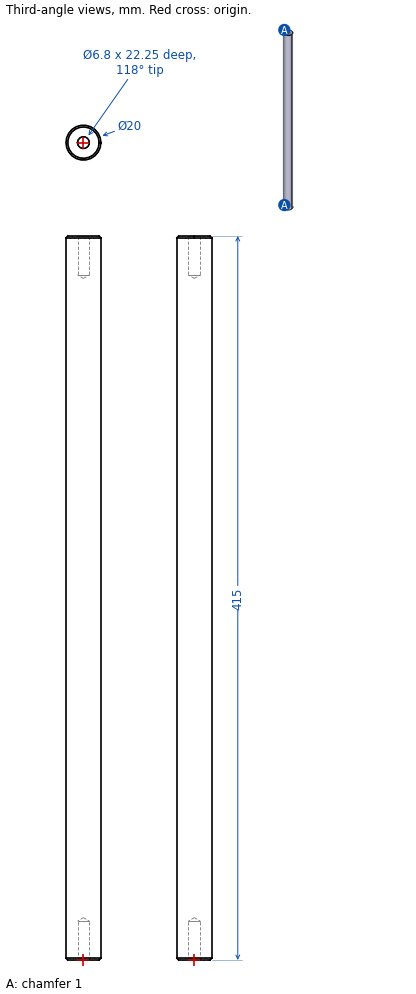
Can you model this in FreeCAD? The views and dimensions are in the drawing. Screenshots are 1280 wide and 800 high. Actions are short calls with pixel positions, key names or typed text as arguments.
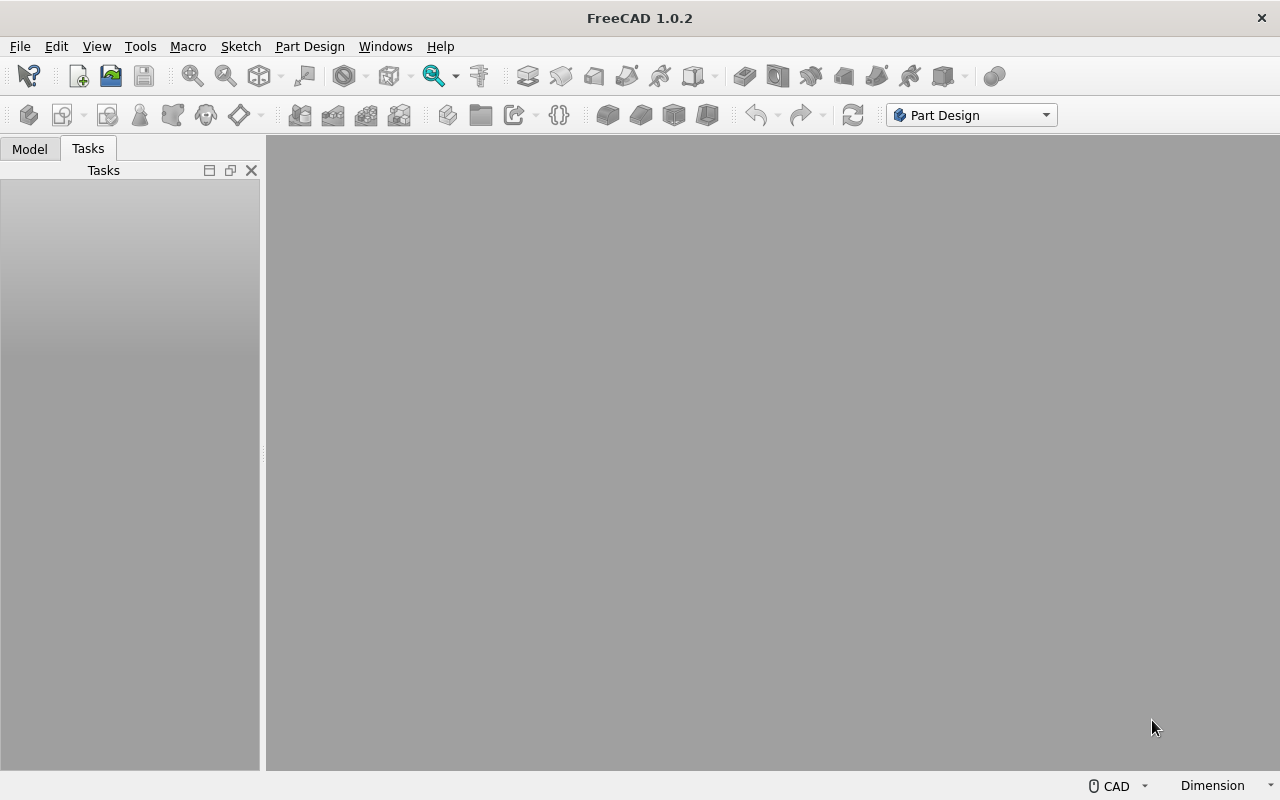
click(78, 76)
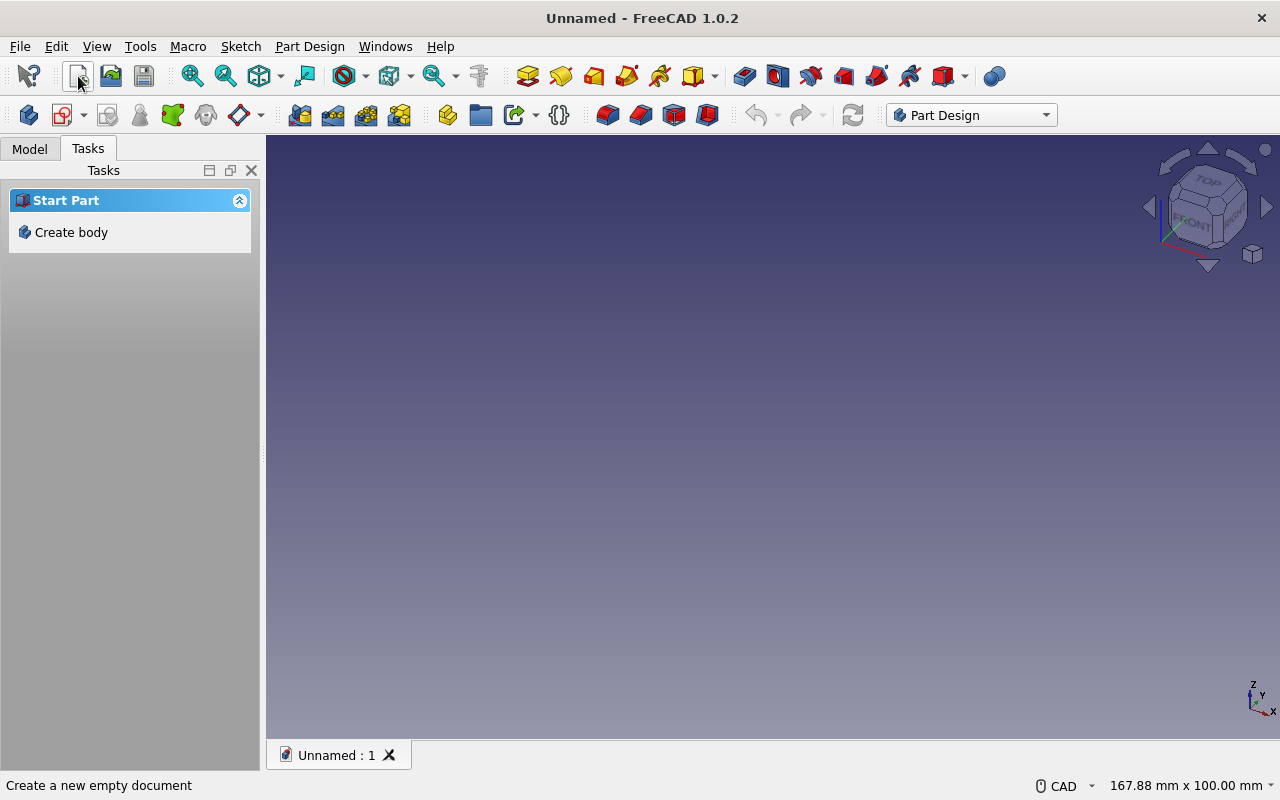
click(62, 116)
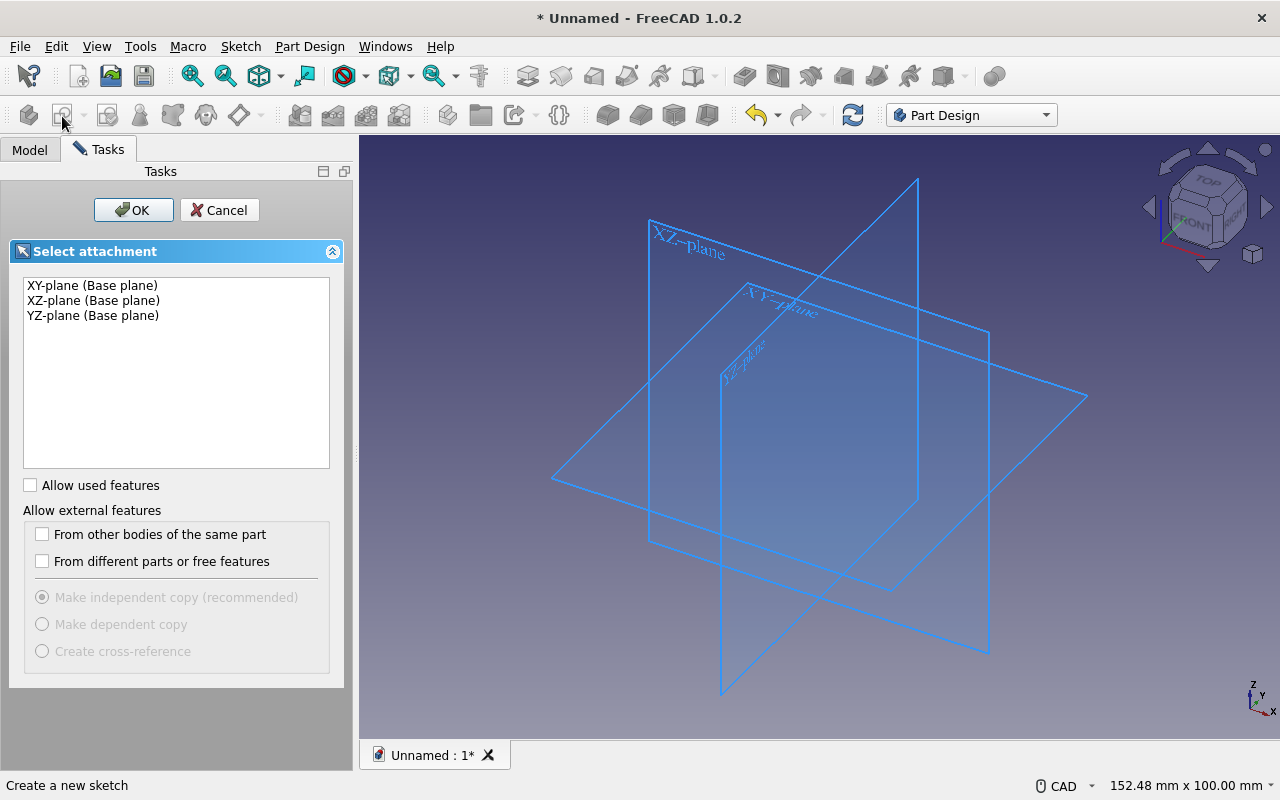
click(84, 286)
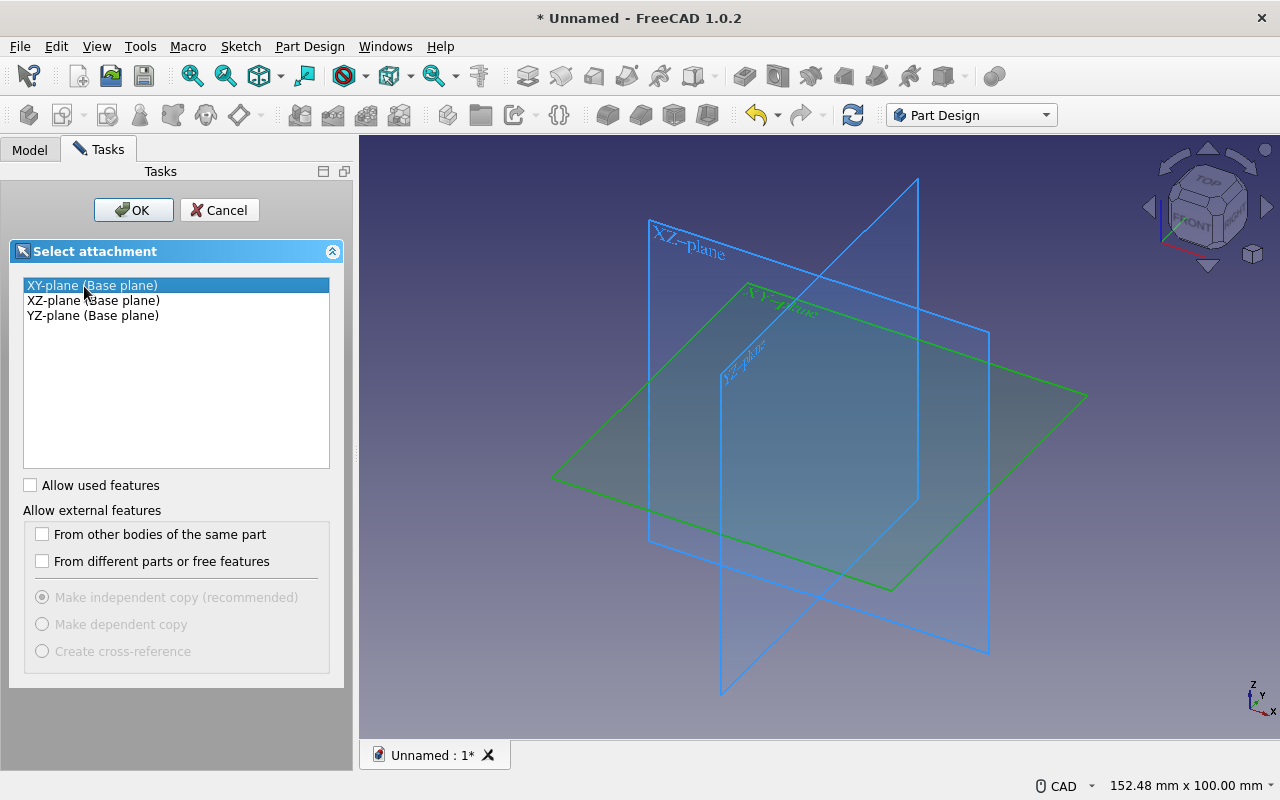
click(134, 210)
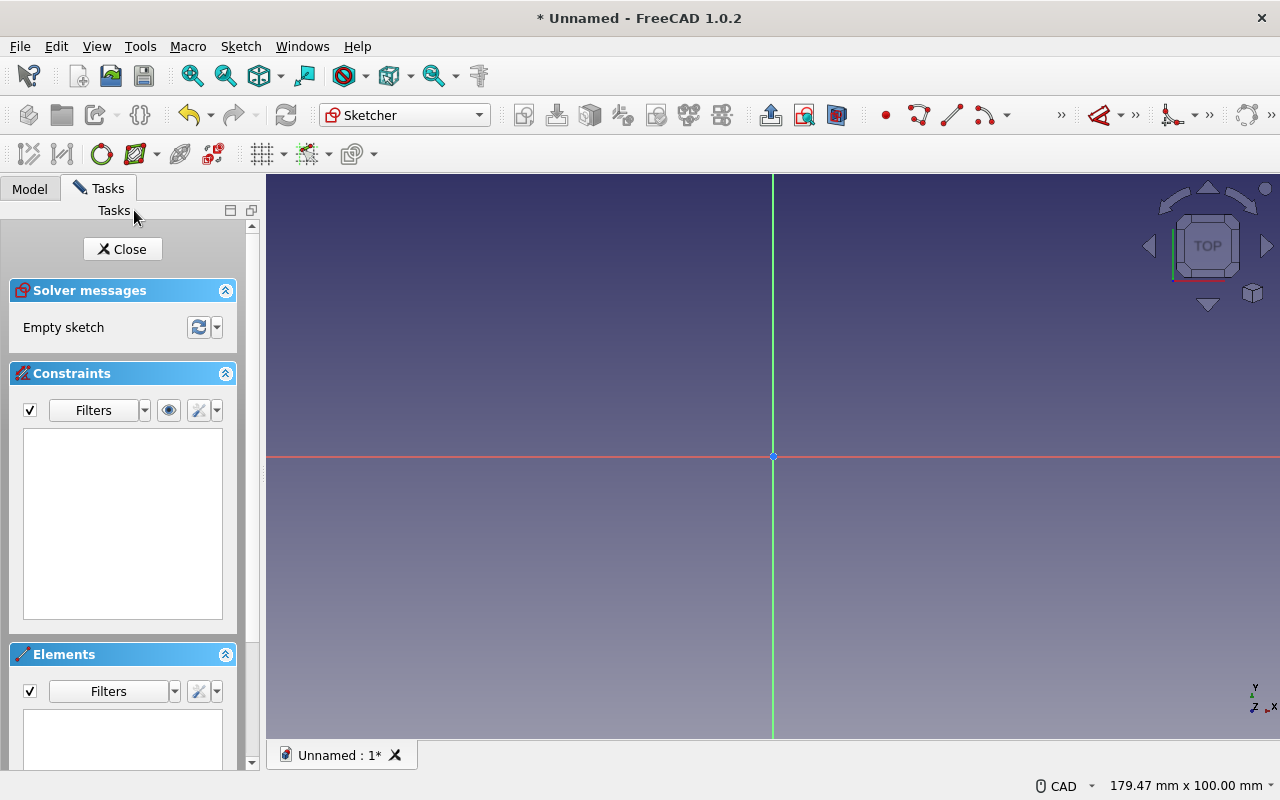
scroll(803, 456, up, 6)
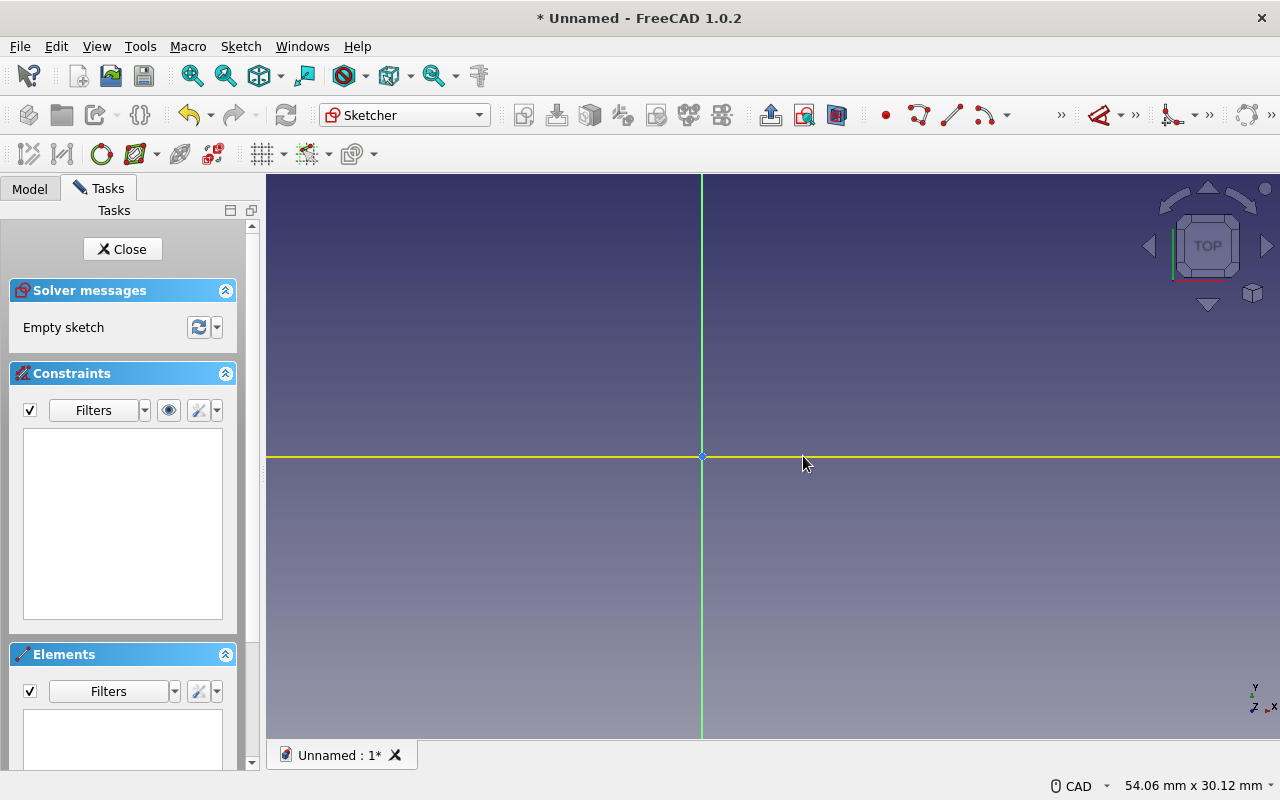
key(g)
key(c)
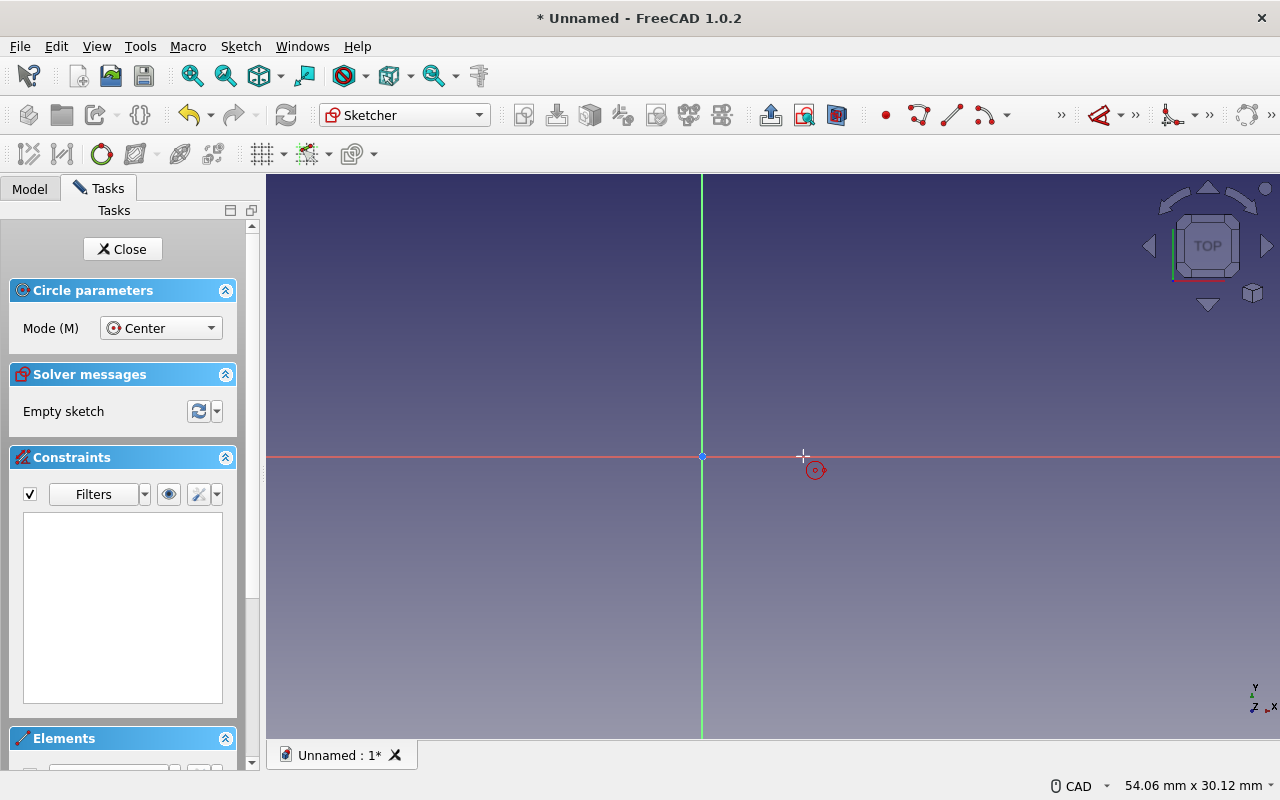
click(702, 456)
click(835, 324)
key(Escape)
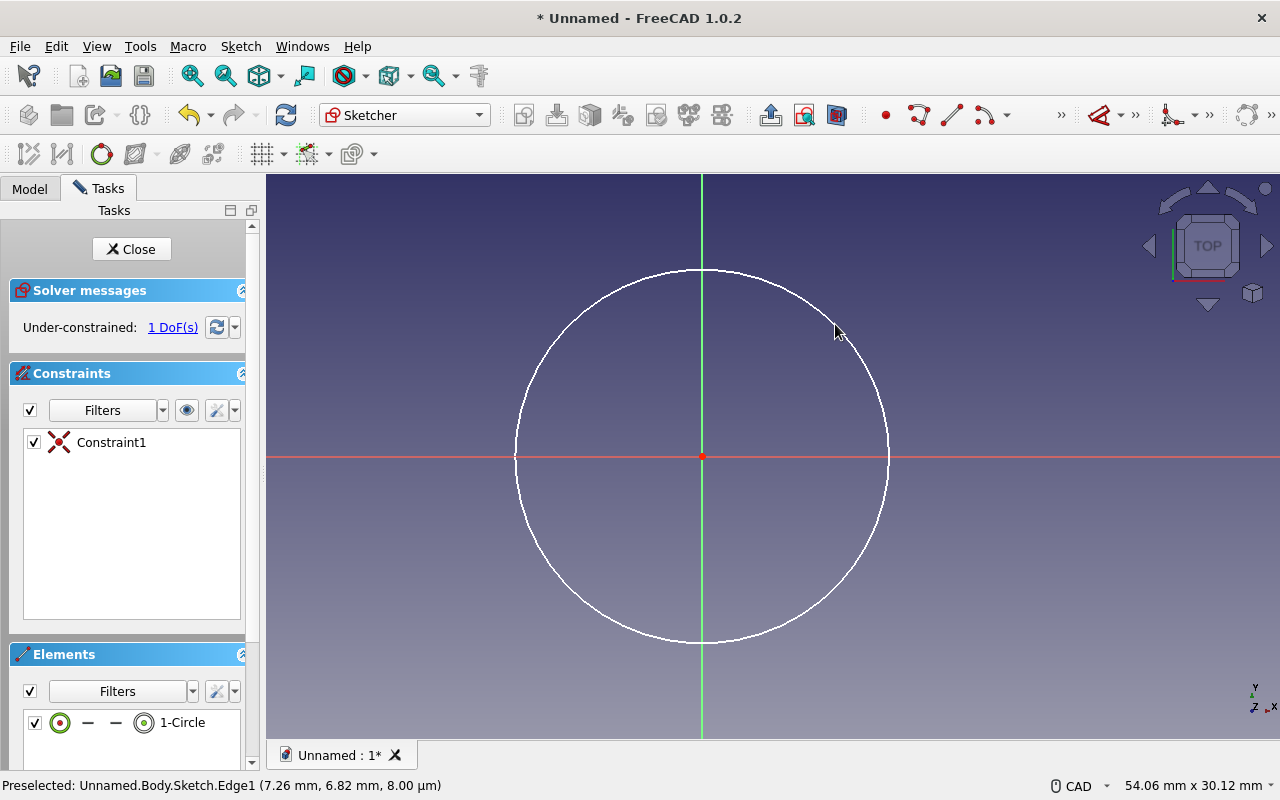
click(834, 324)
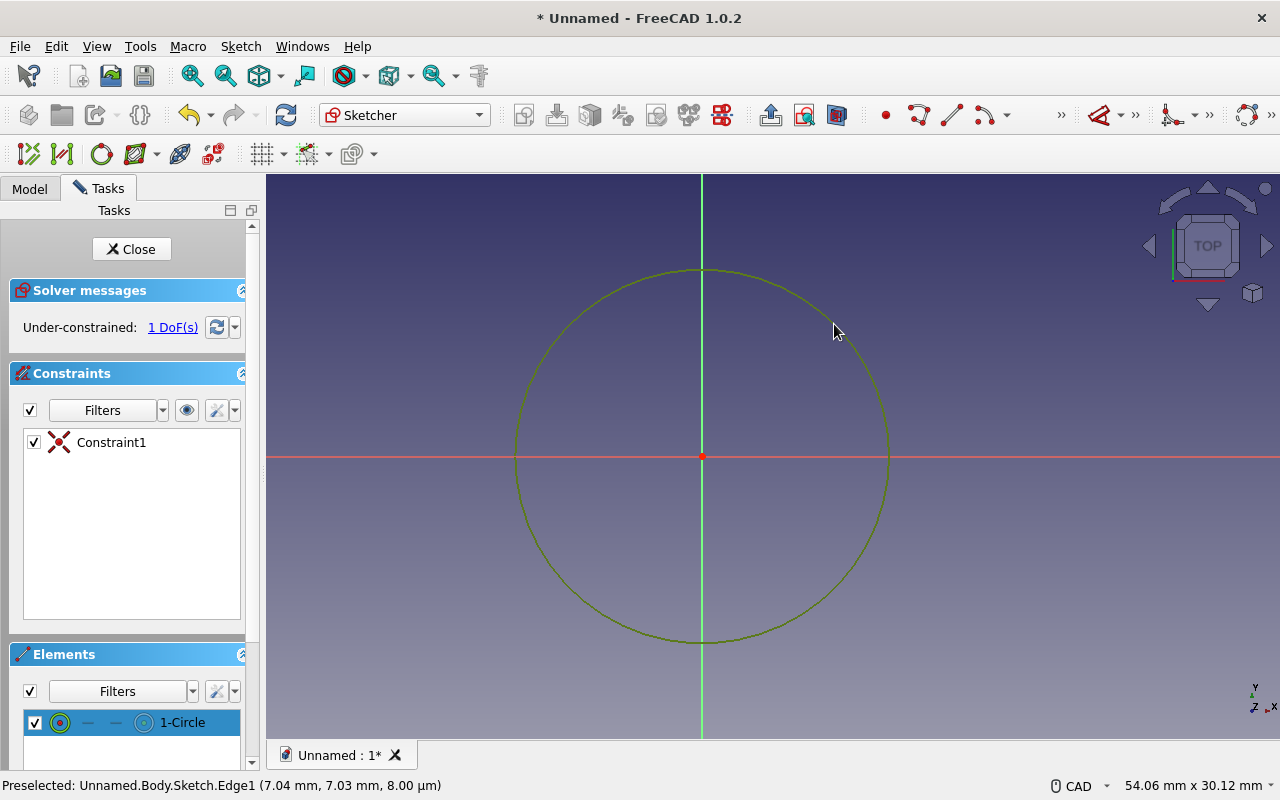
click(1120, 116)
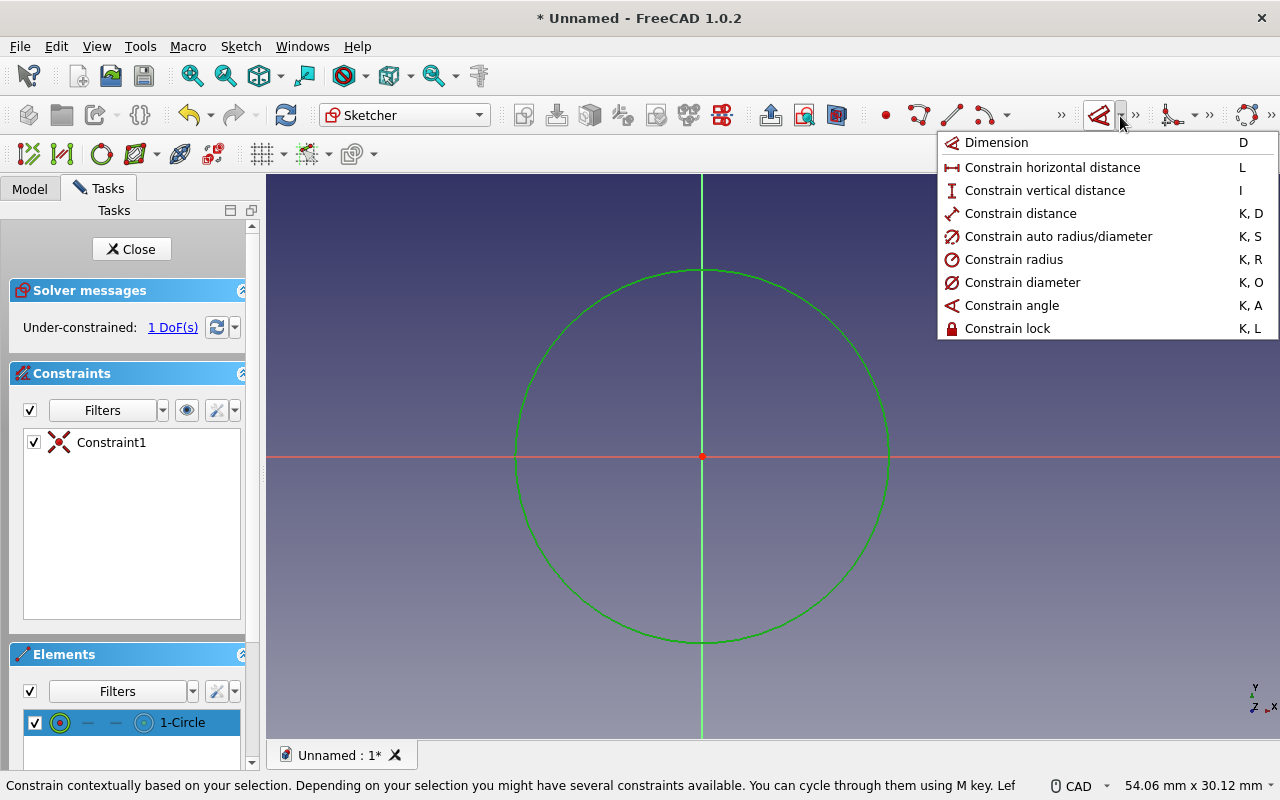
click(1108, 282)